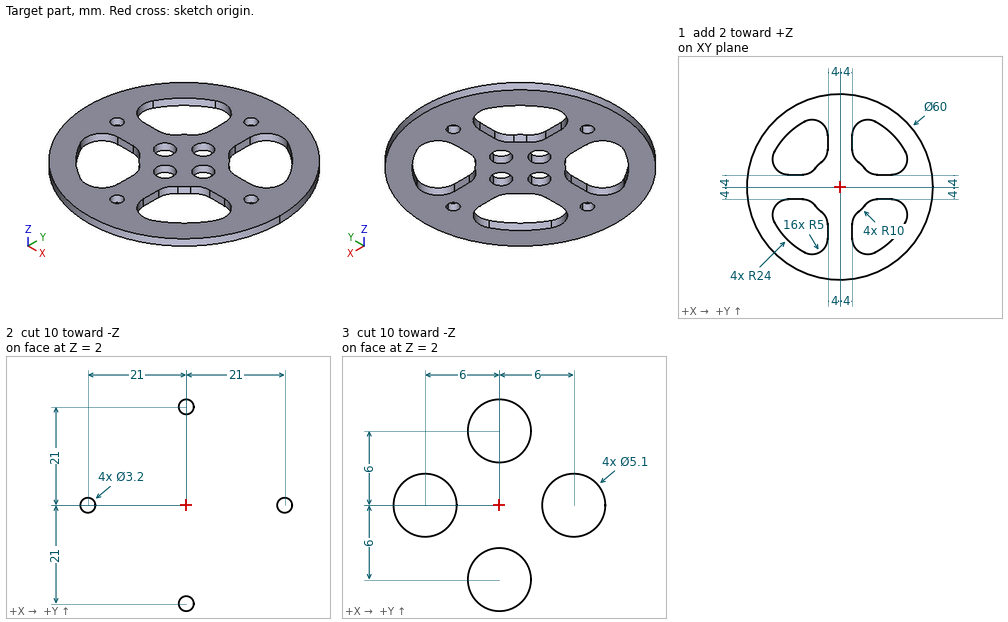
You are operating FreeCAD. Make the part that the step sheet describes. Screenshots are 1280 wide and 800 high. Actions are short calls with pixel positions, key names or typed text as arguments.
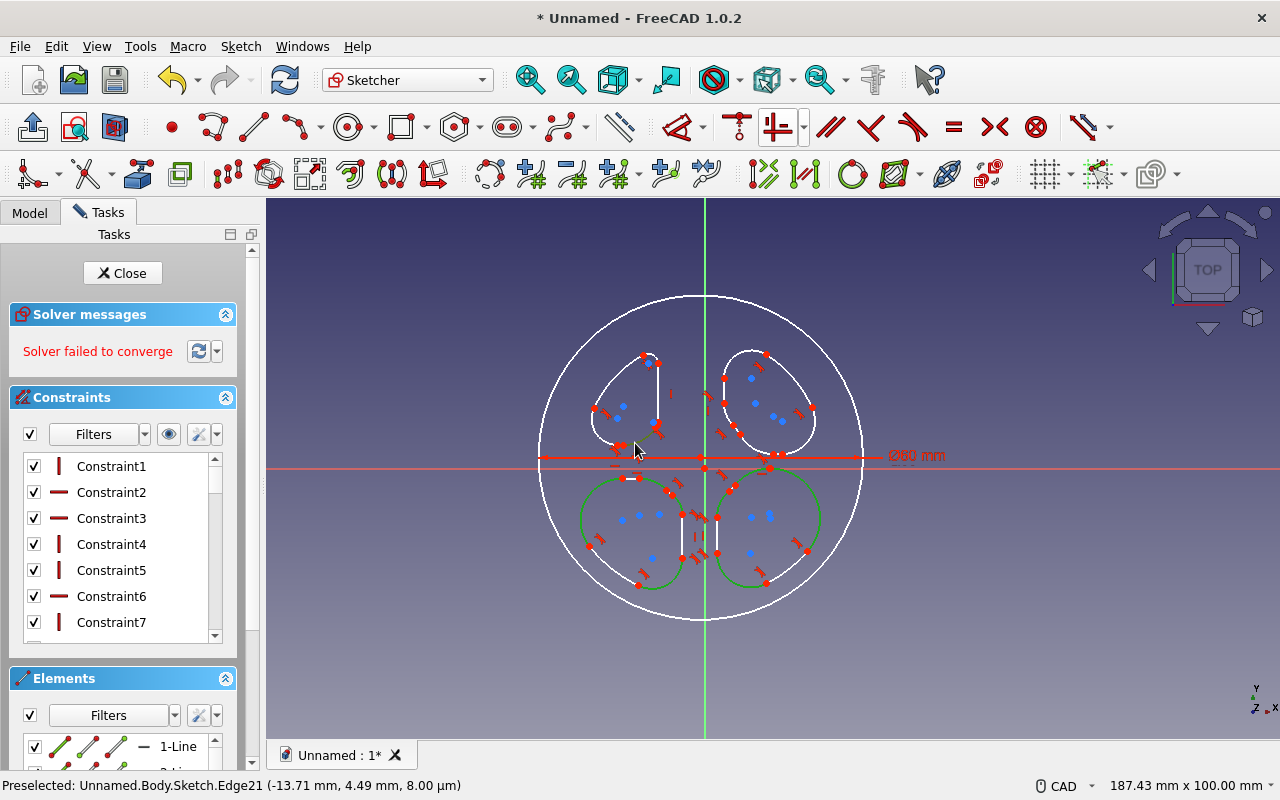
click(592, 423)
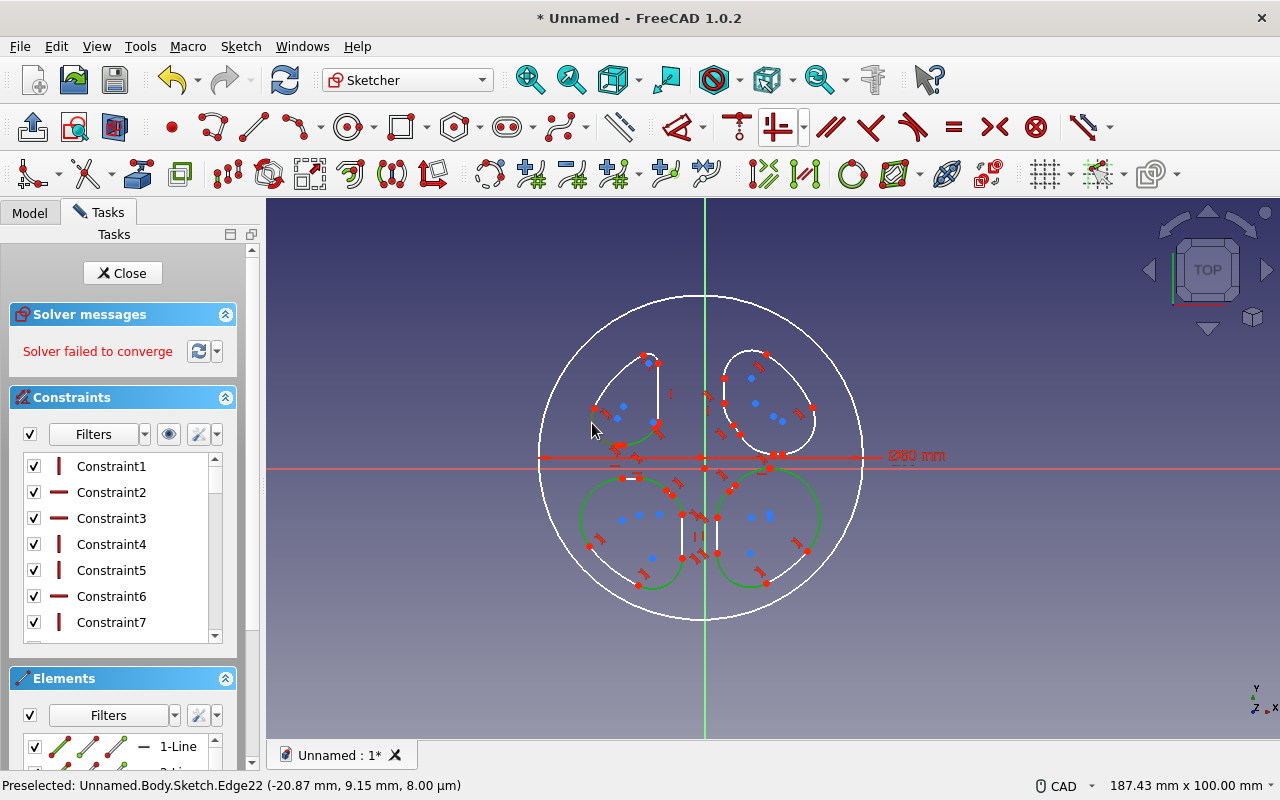
scroll(653, 355, up, 2)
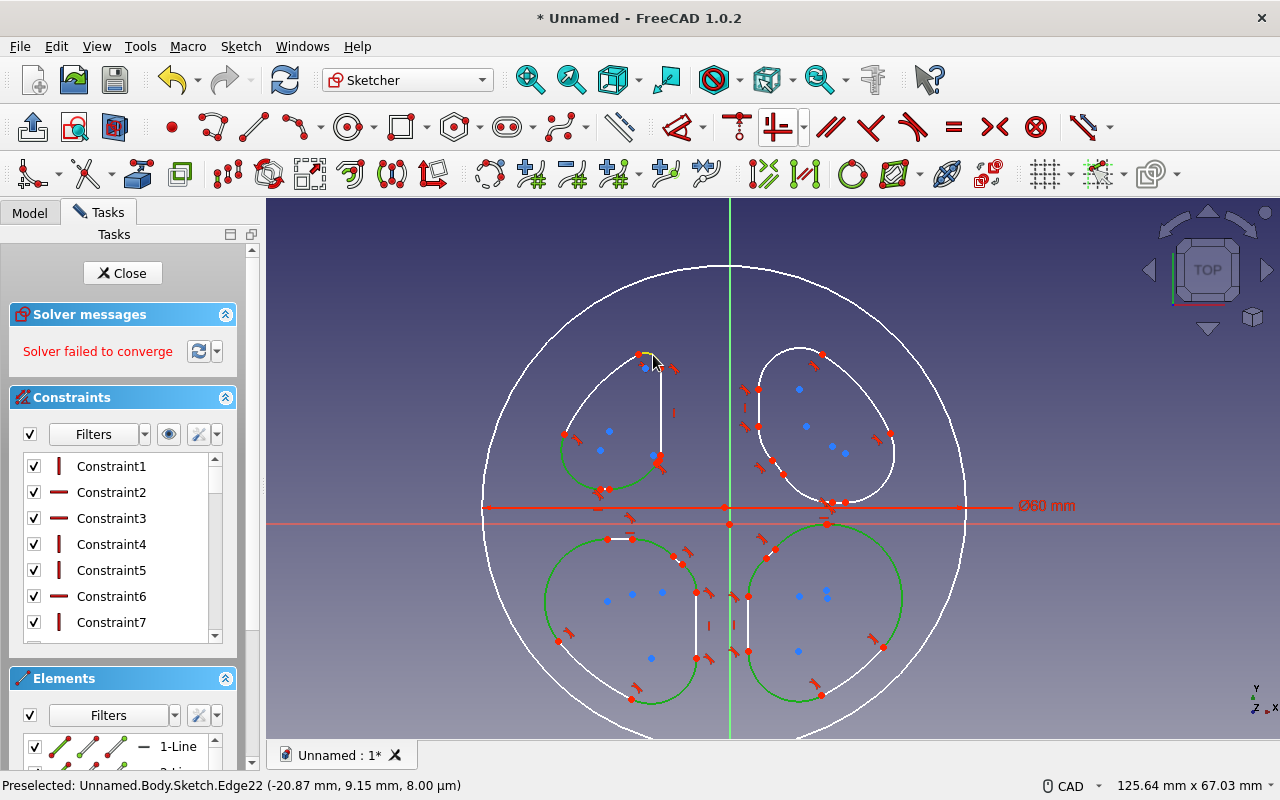
click(653, 355)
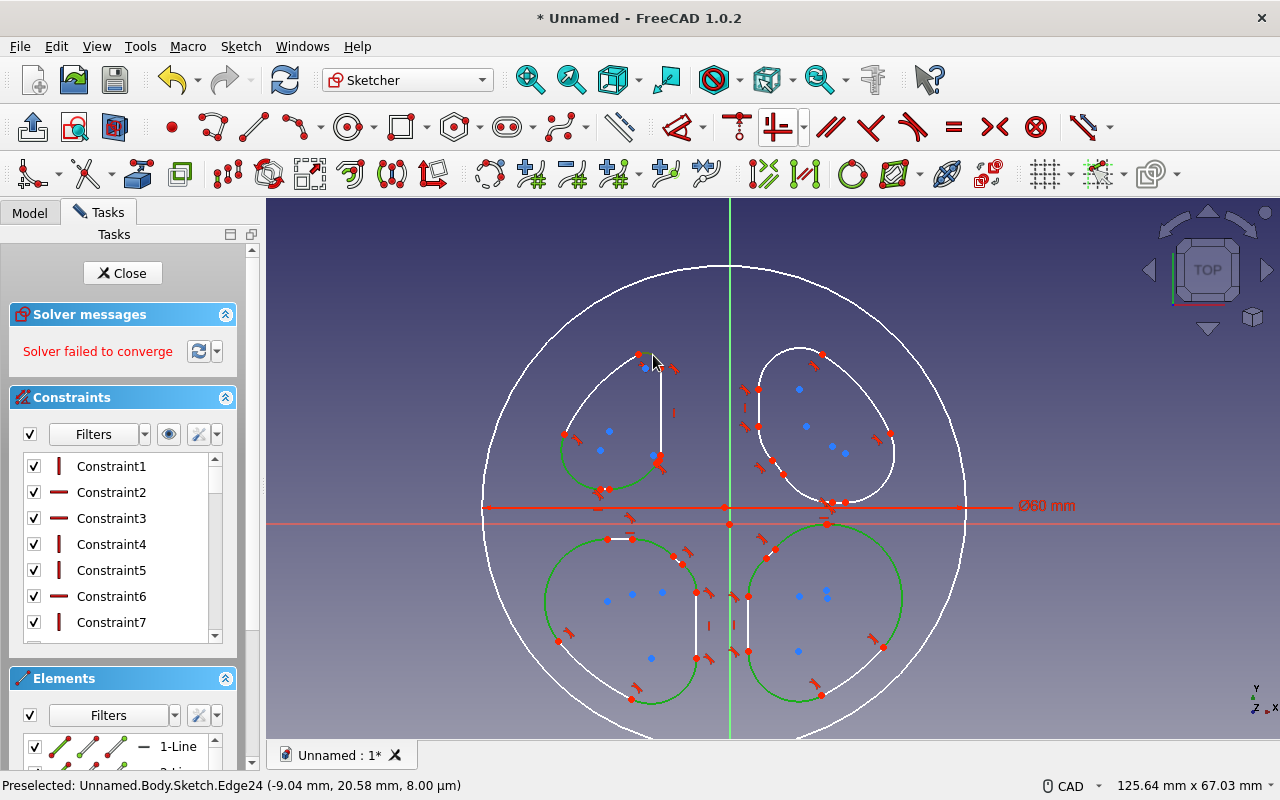
click(797, 348)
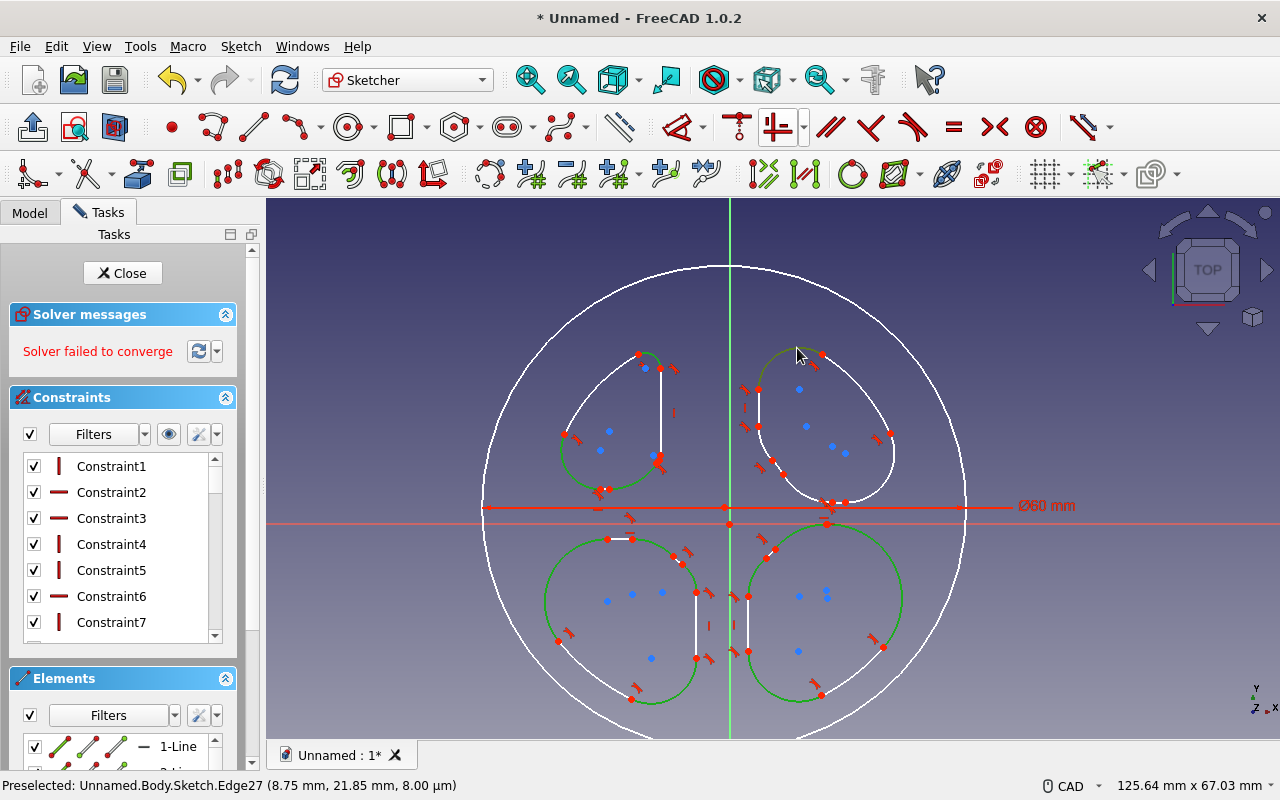
click(873, 494)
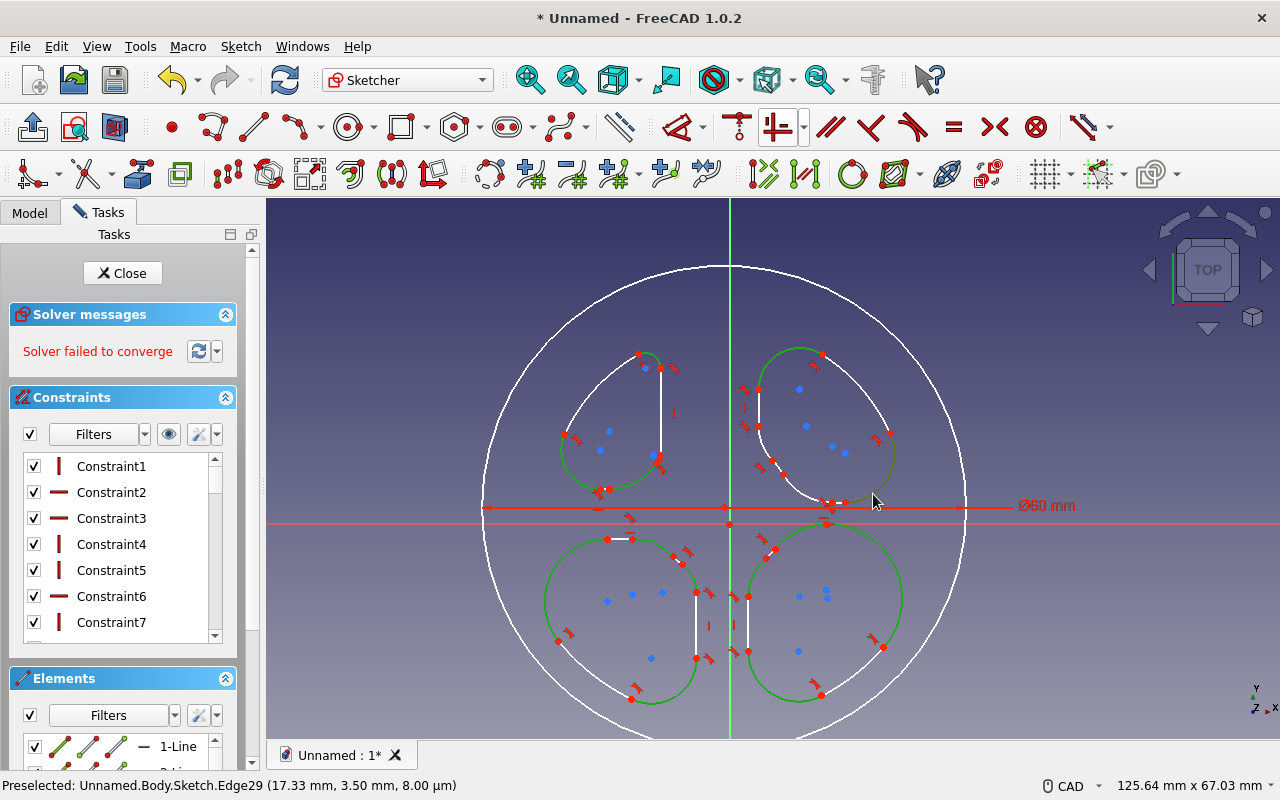
click(794, 488)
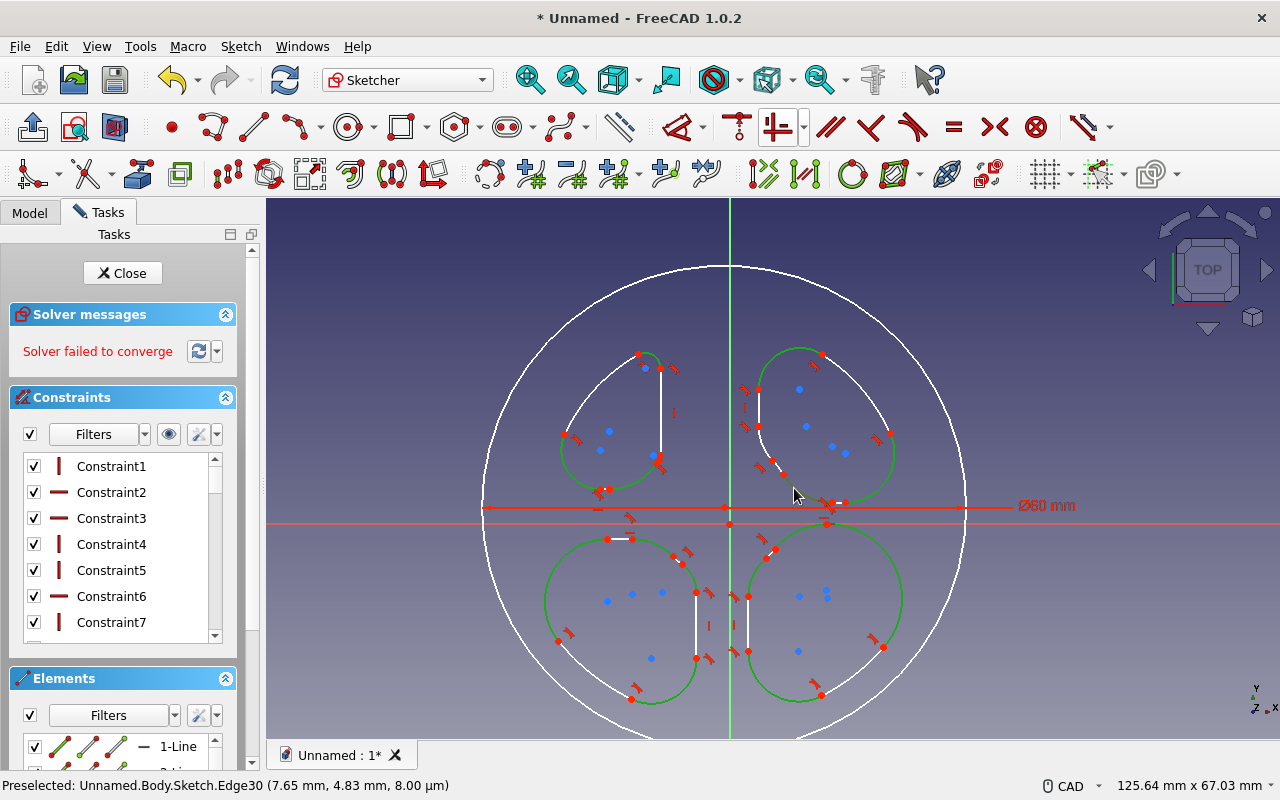
scroll(760, 438, up, 2)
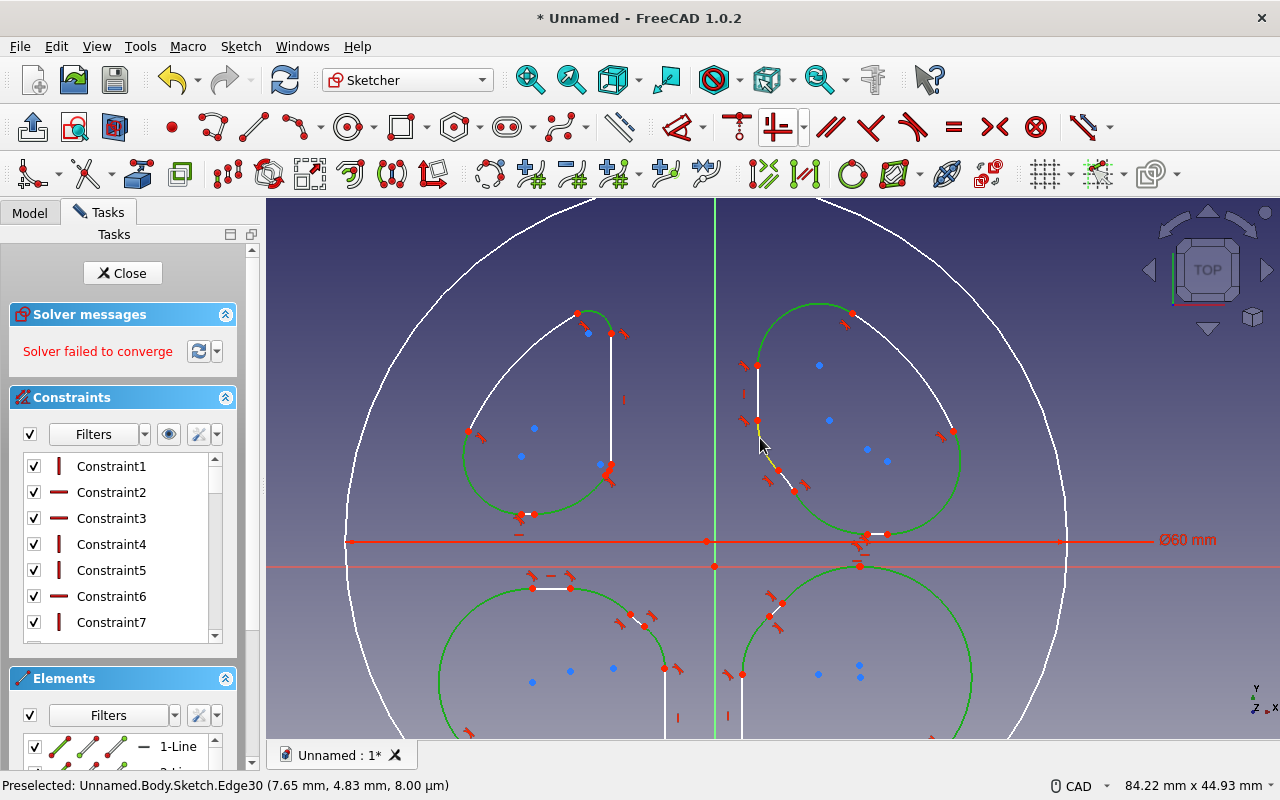
click(760, 437)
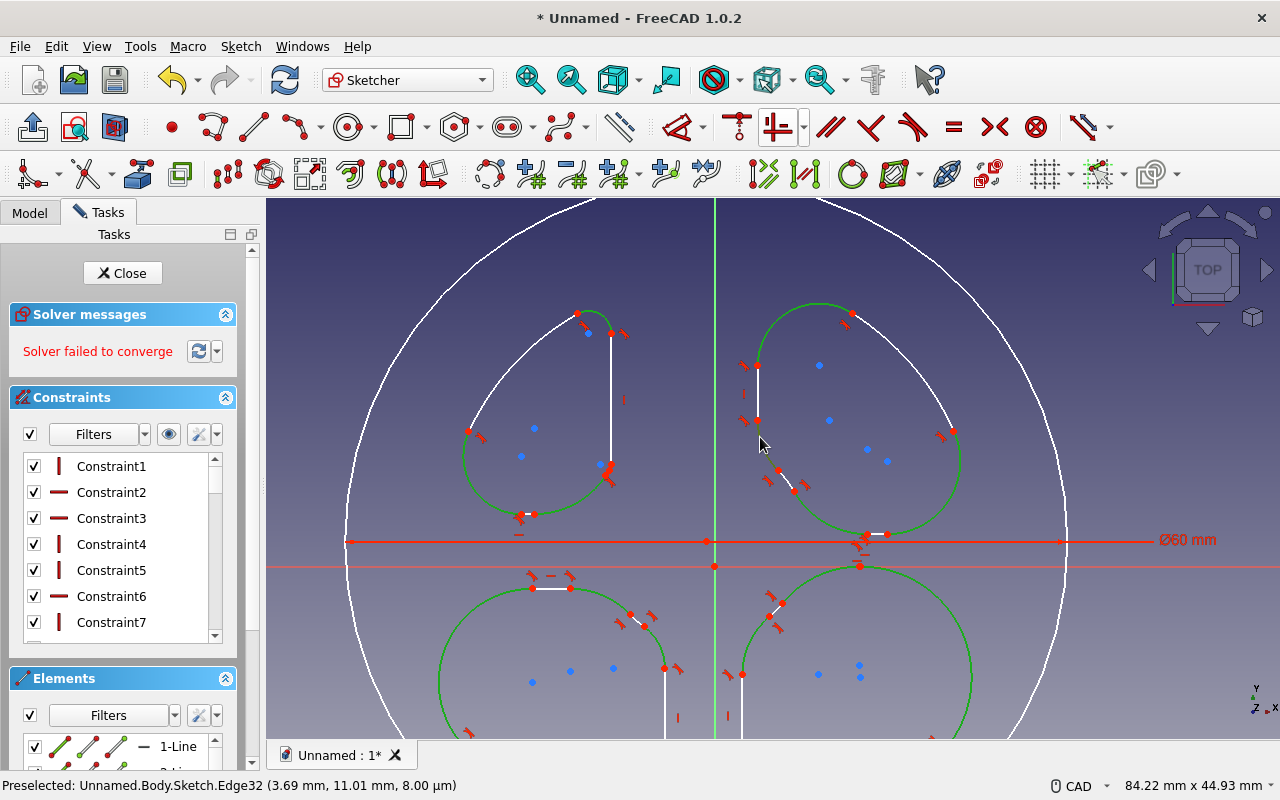
click(954, 128)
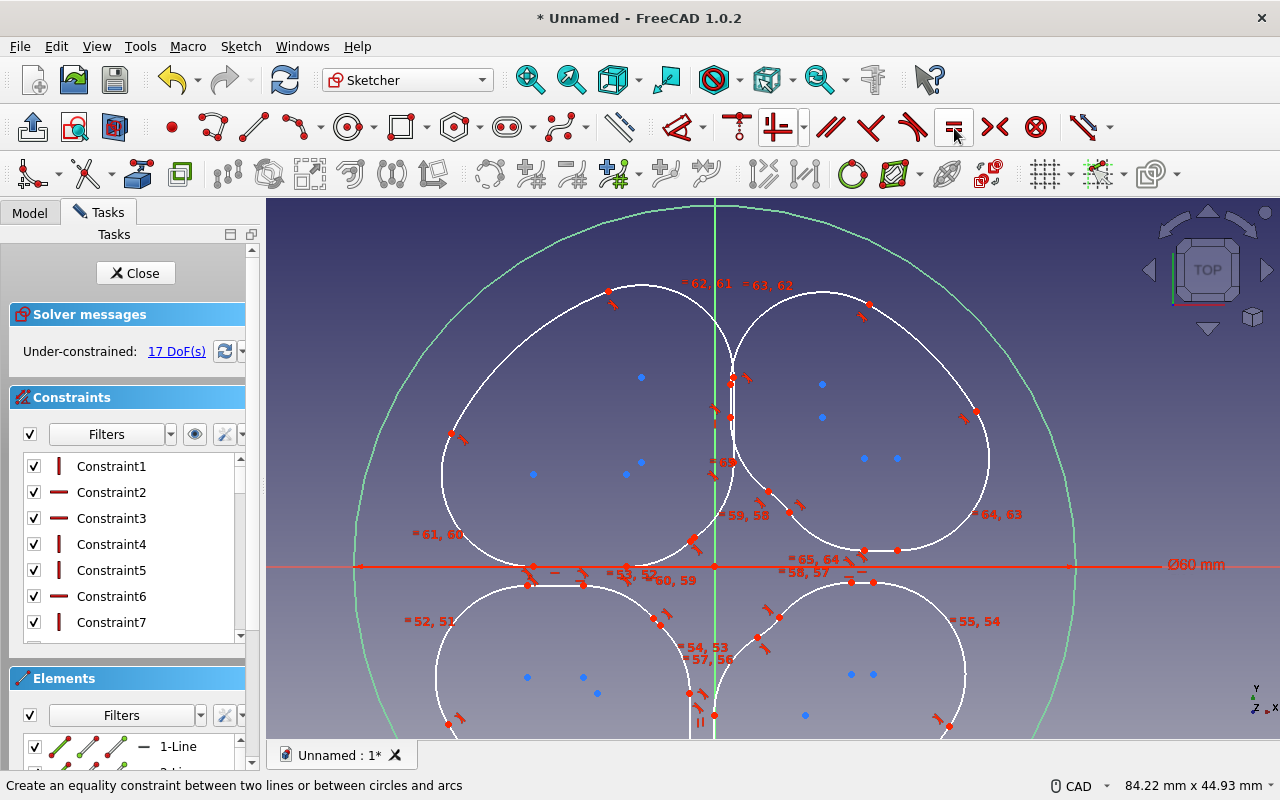
scroll(696, 388, down, 4)